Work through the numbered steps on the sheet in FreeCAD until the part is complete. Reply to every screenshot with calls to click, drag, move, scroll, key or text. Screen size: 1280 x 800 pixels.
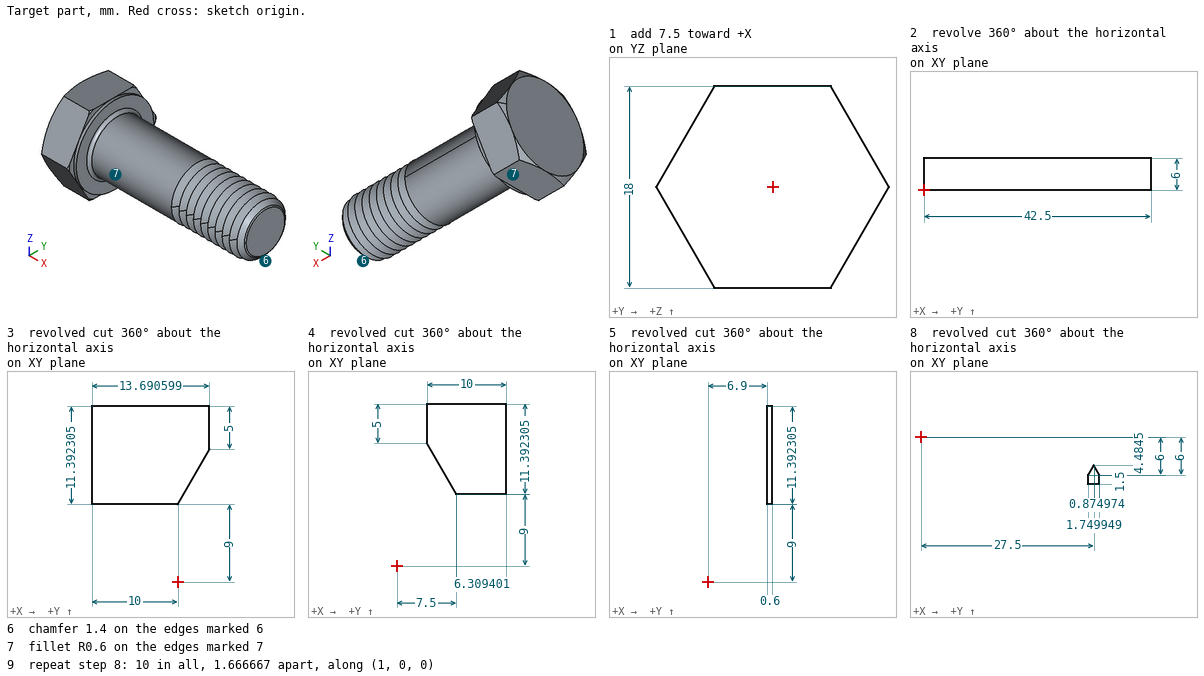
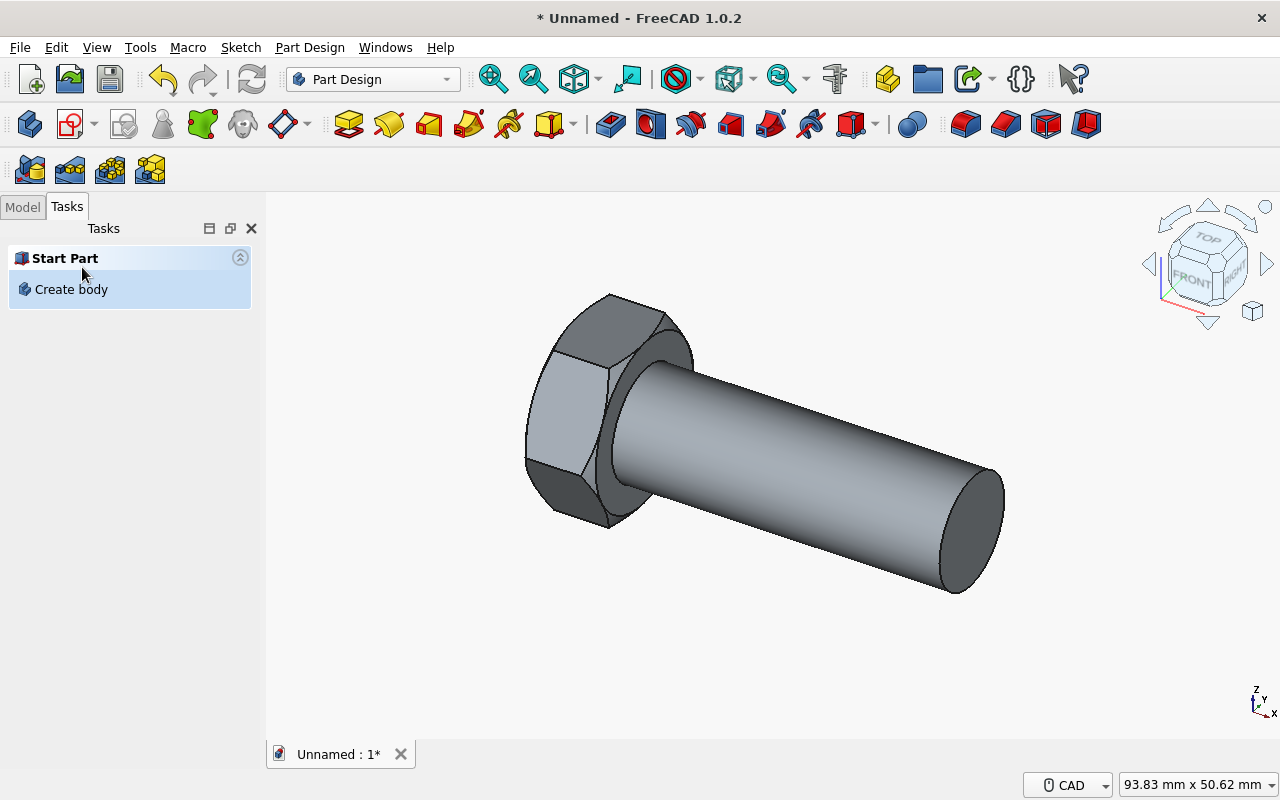
click(70, 124)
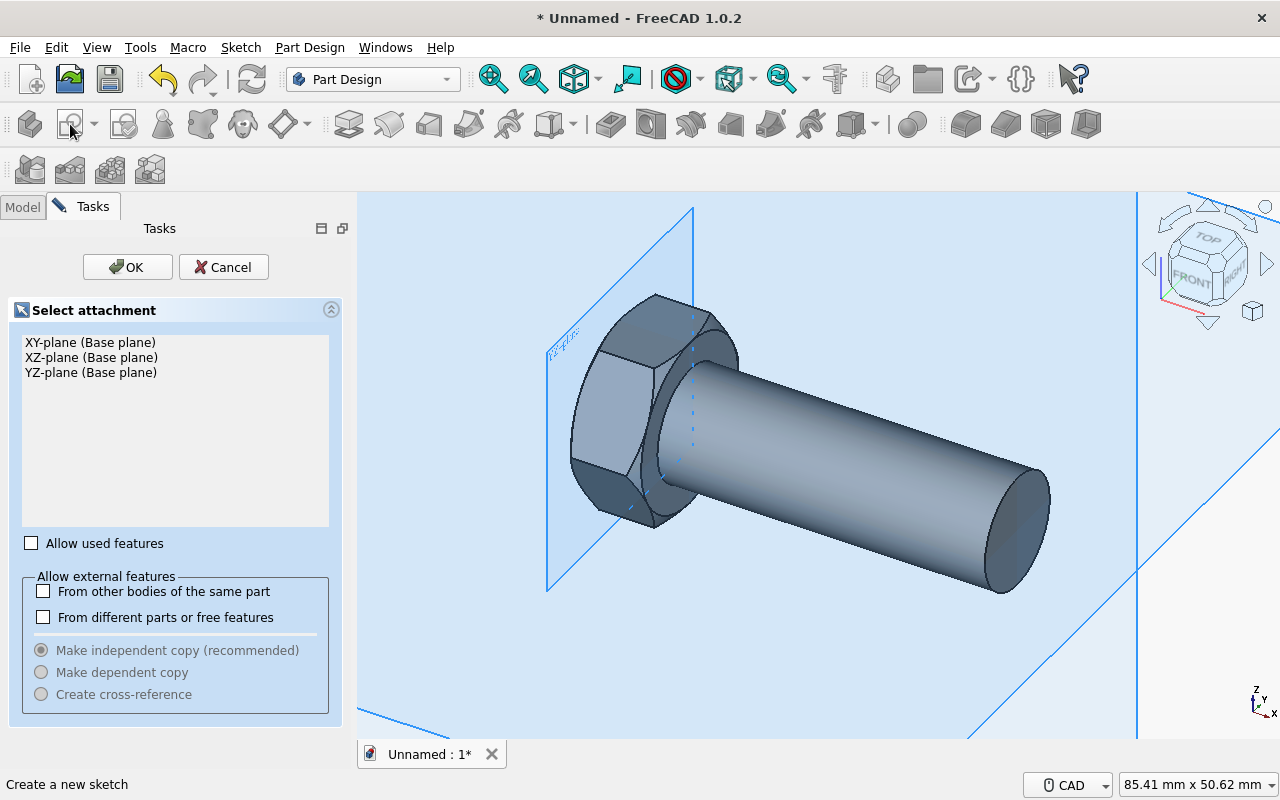
click(82, 342)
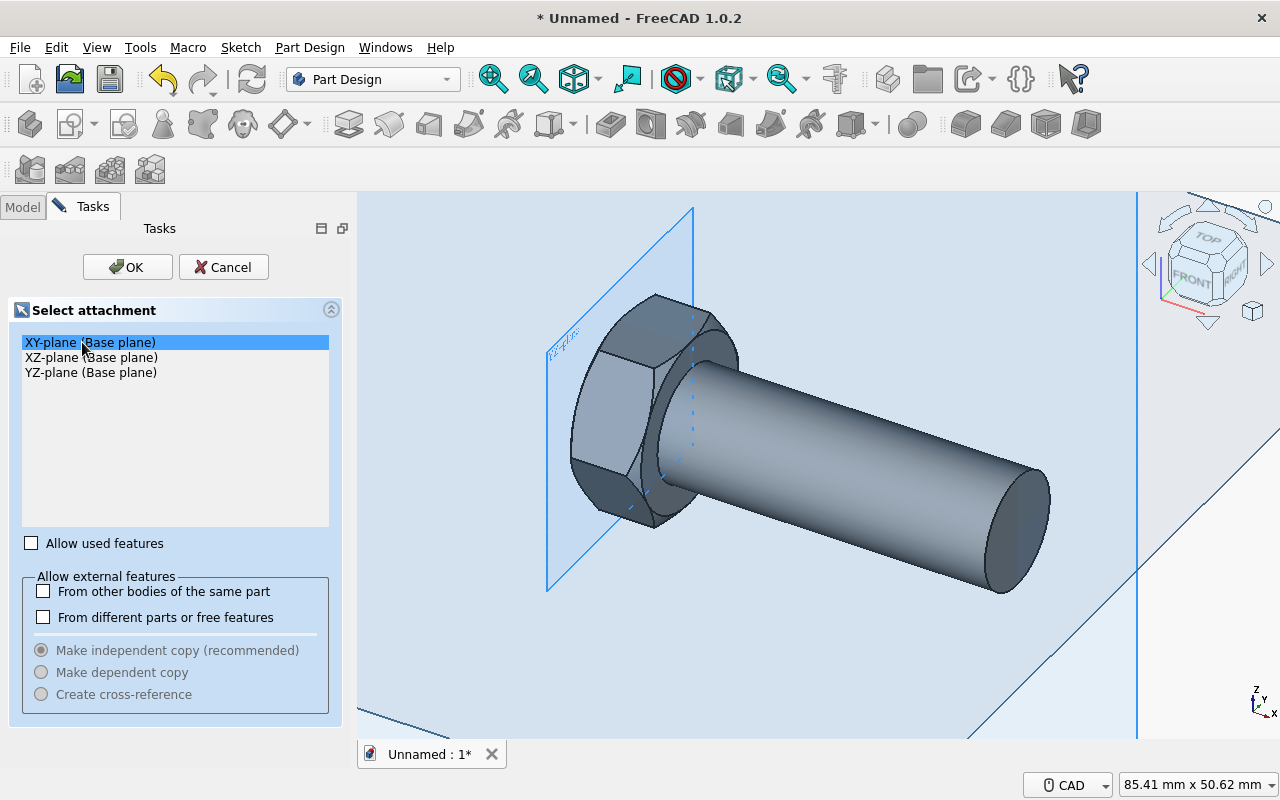
click(128, 267)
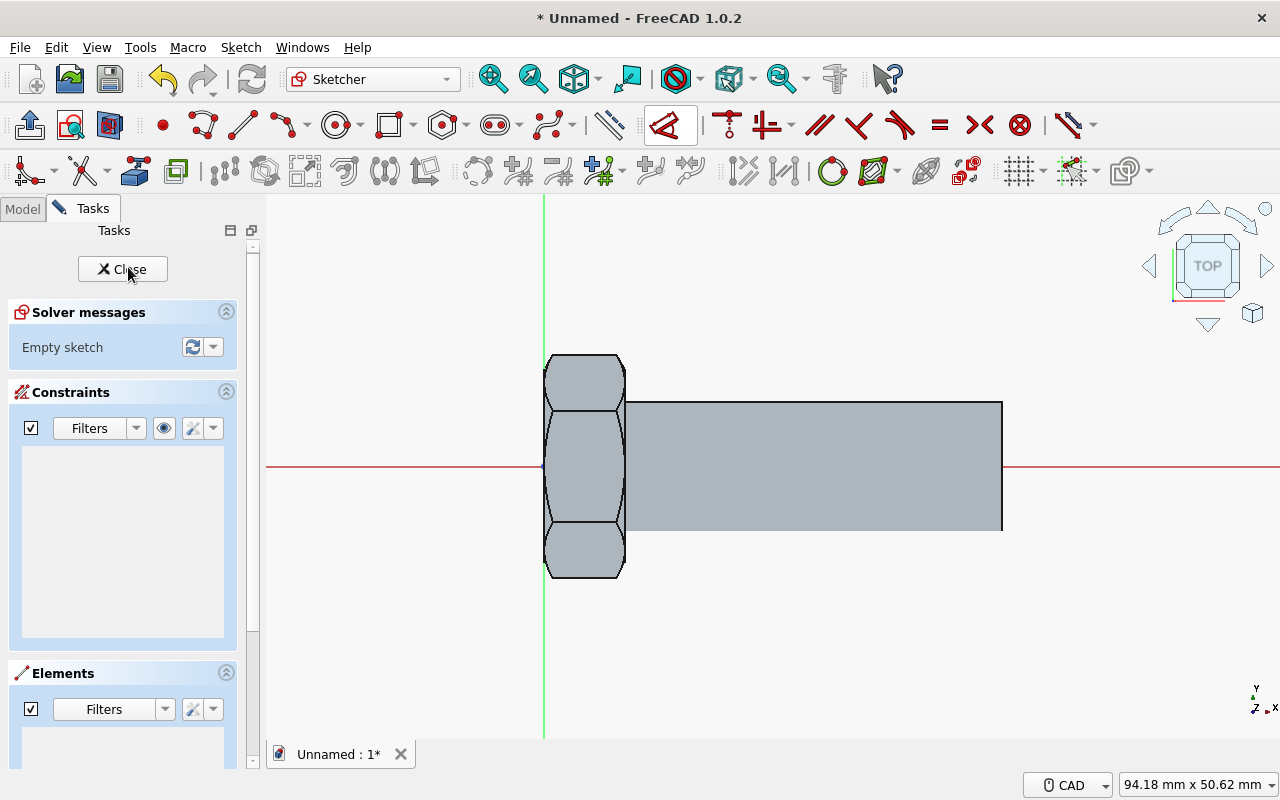
key(q)
key(s)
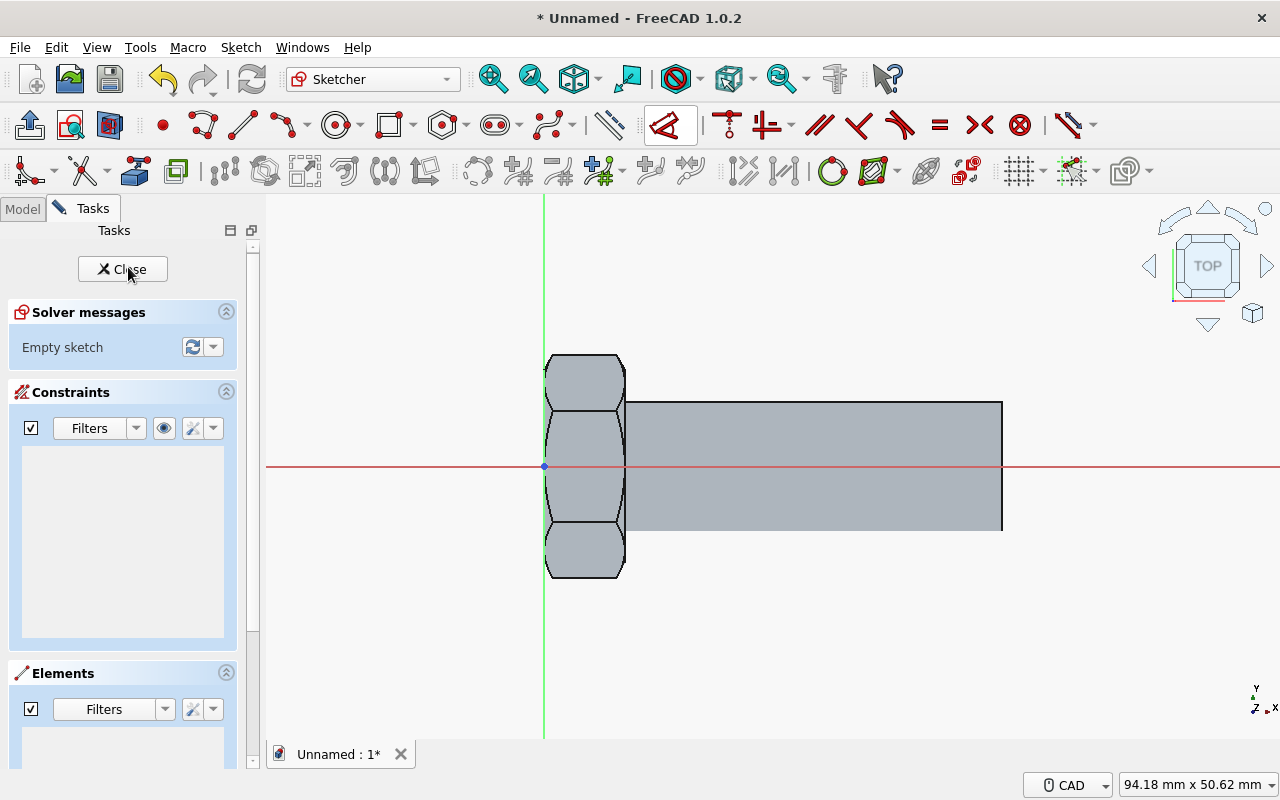
scroll(341, 222, up, 2)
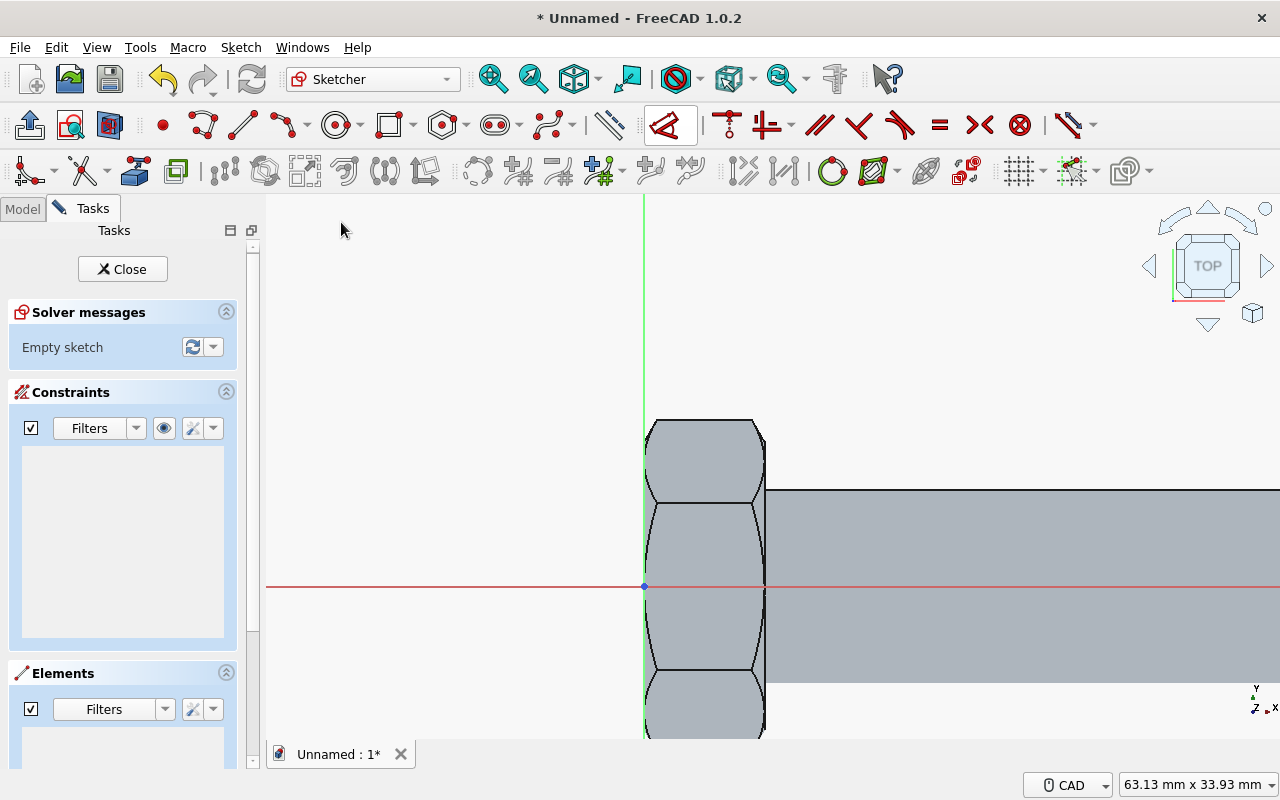
key(g)
key(r)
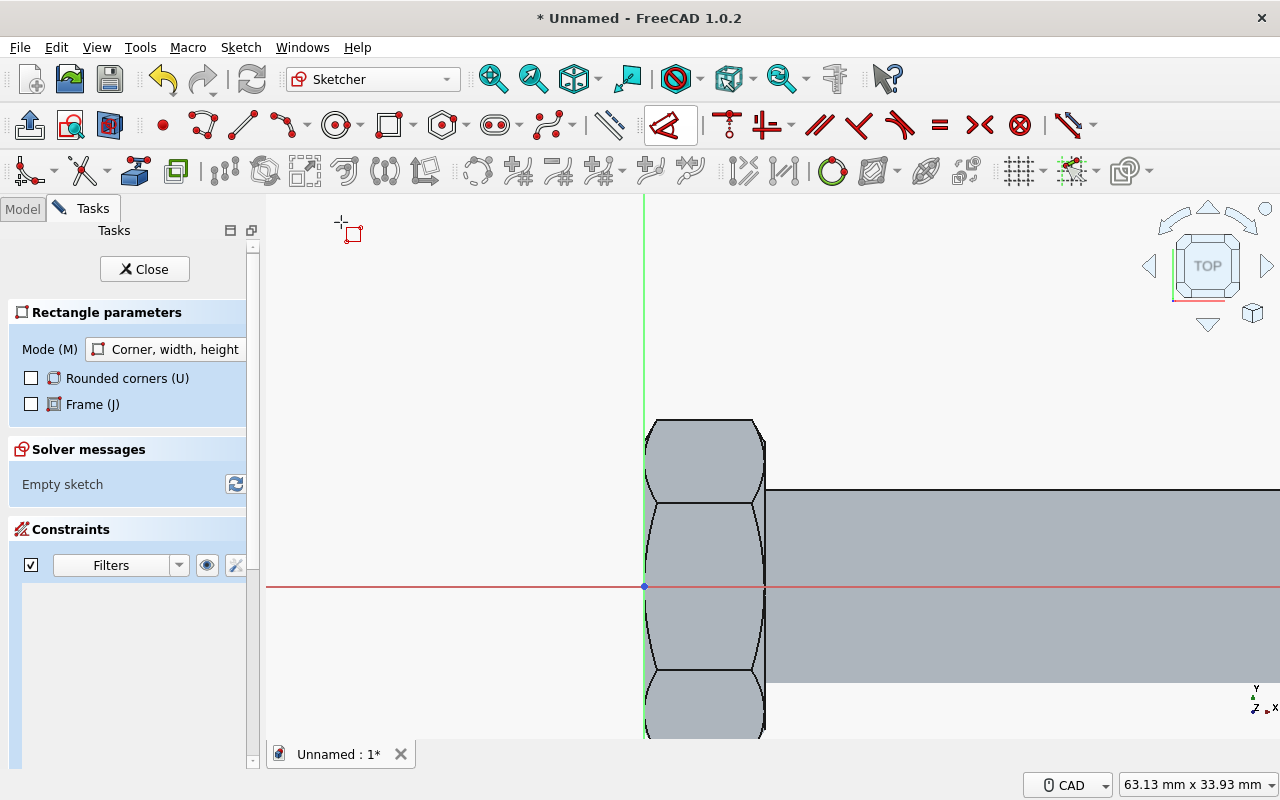
scroll(755, 259, up, 3)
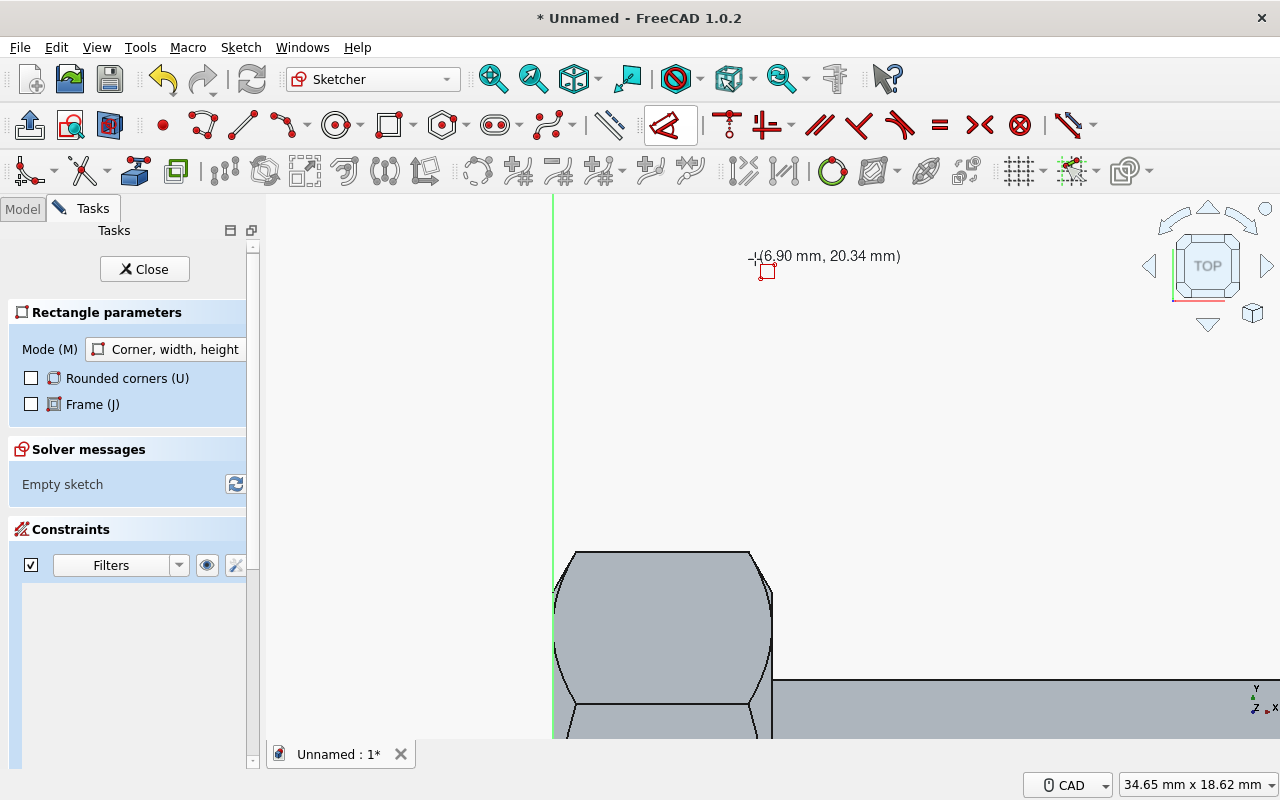
click(754, 259)
click(772, 593)
key(Escape)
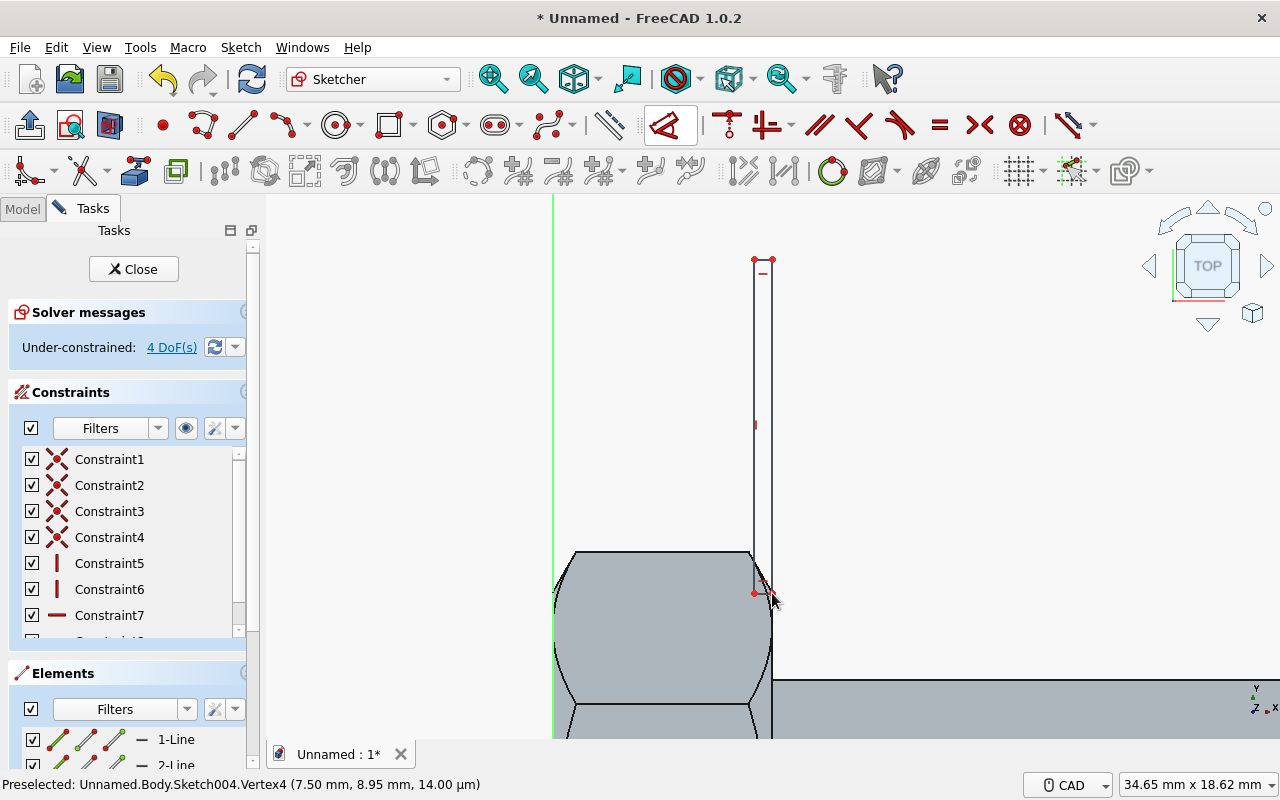
click(754, 594)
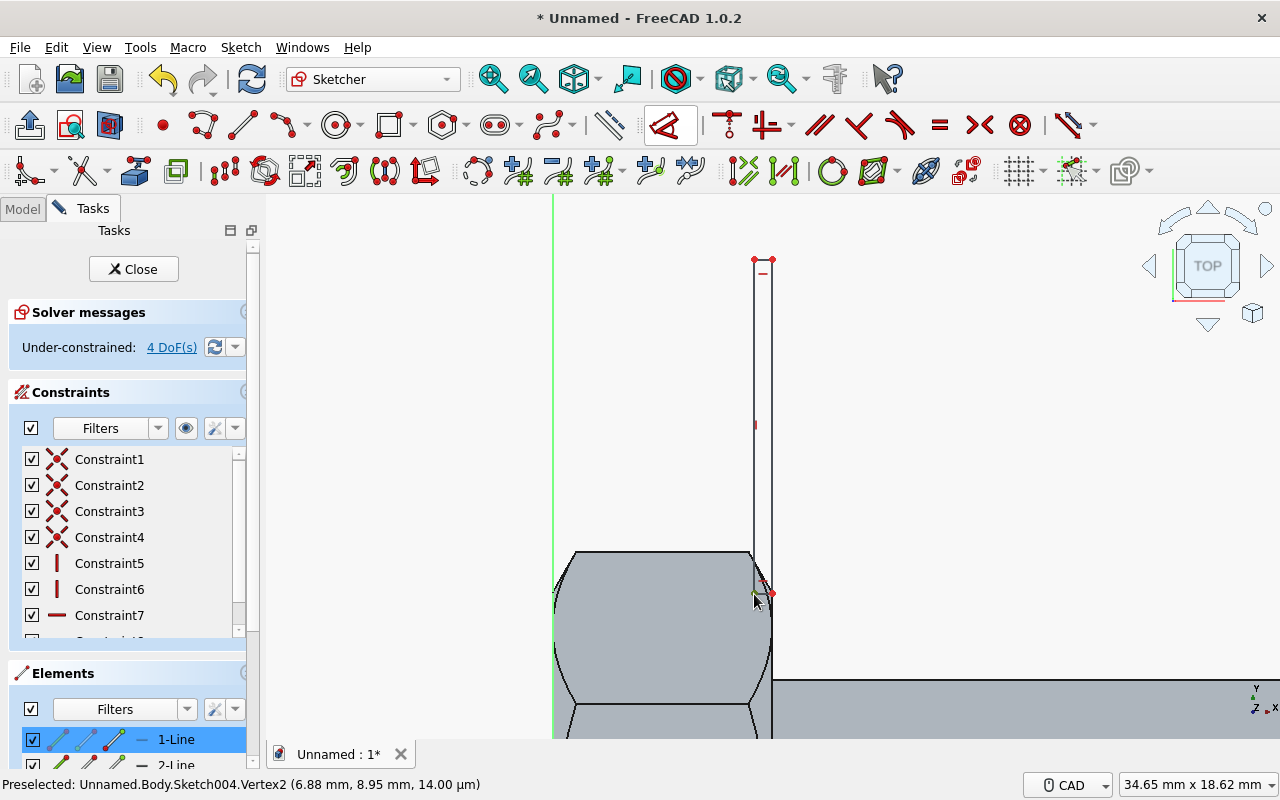
key(i)